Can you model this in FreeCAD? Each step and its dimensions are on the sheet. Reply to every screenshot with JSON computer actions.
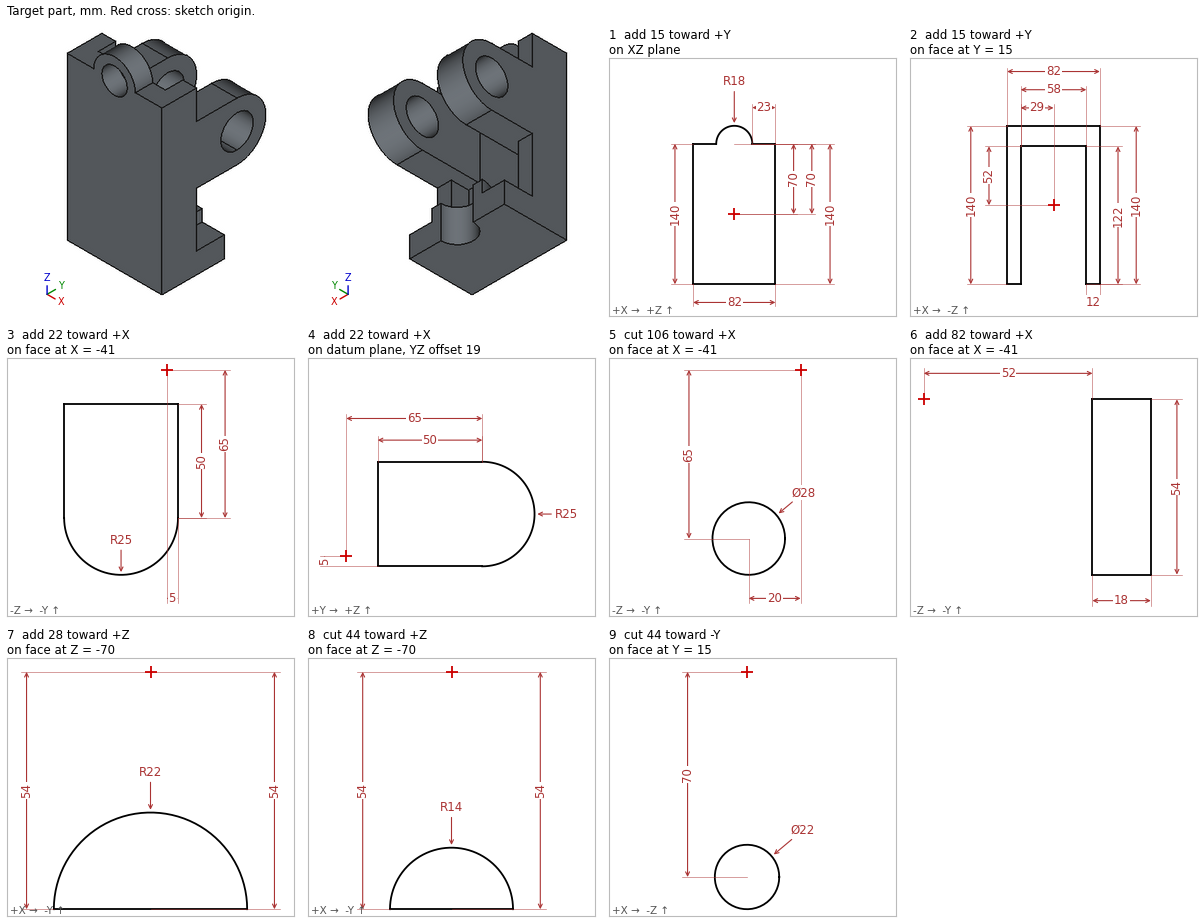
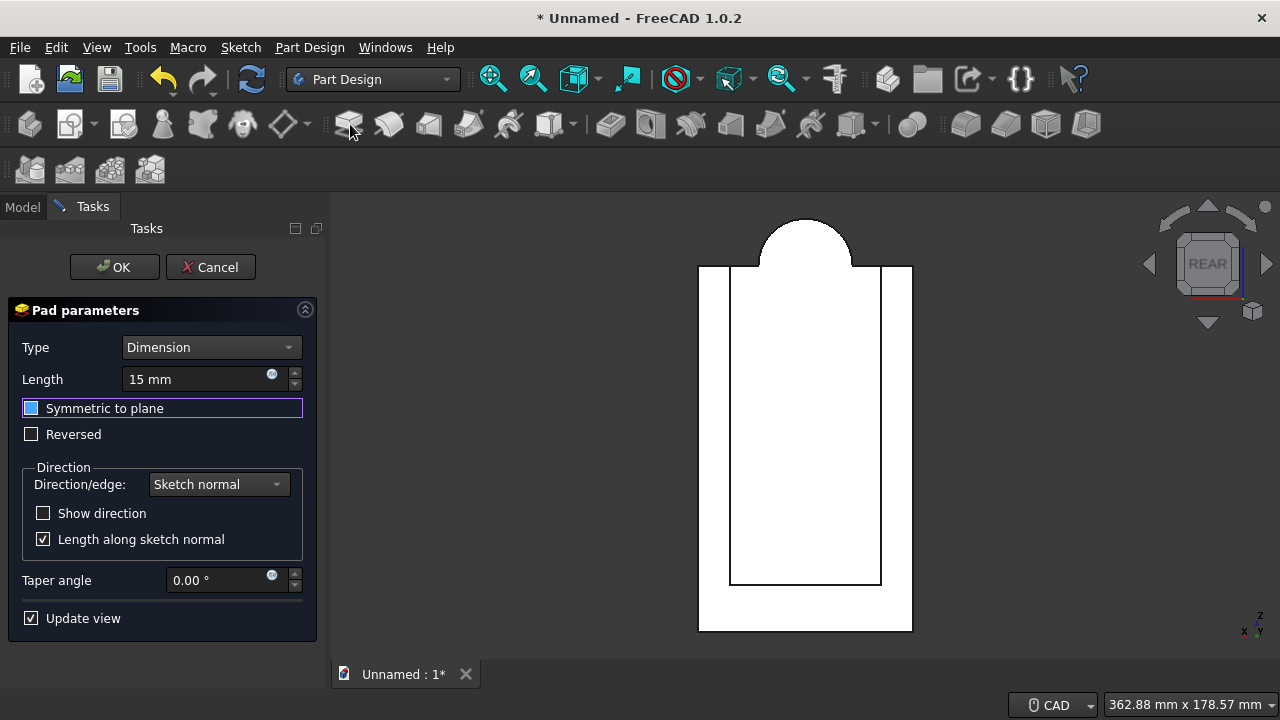
{"action": "left_click", "coordinate": [115, 267]}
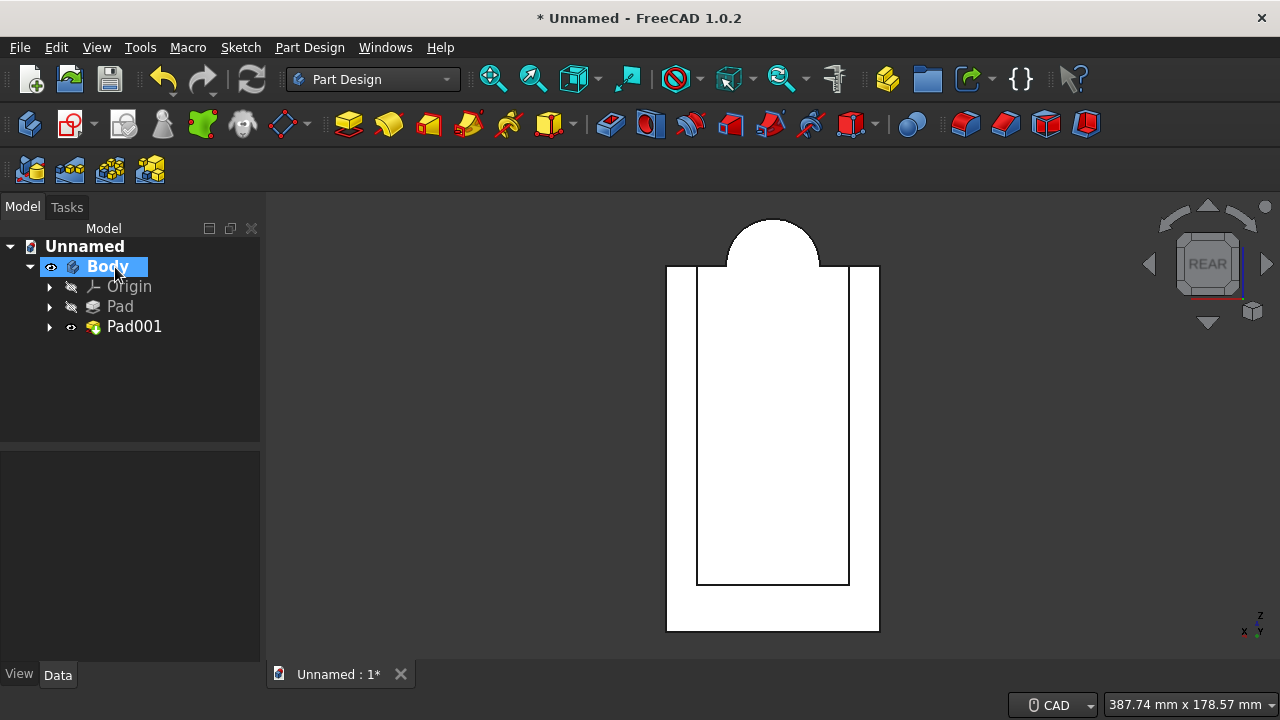
{"action": "key", "text": "6"}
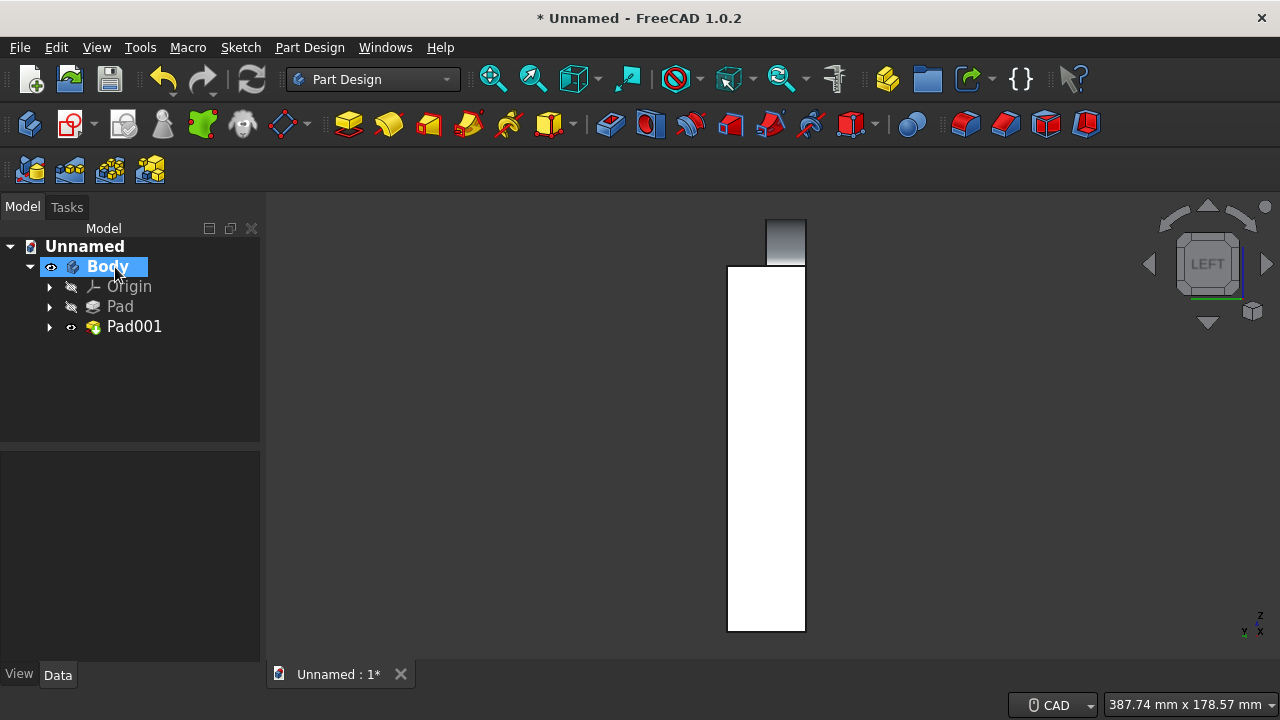
{"action": "left_click", "coordinate": [766, 553]}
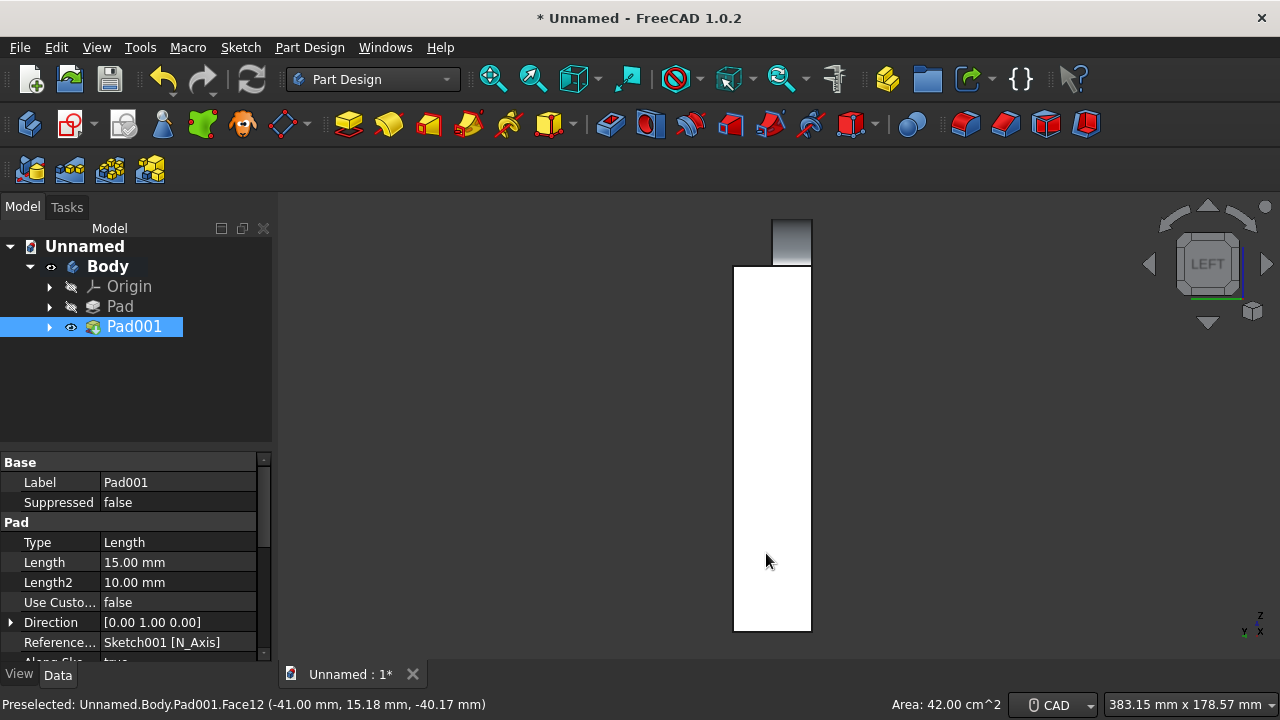
{"action": "left_click", "coordinate": [70, 124]}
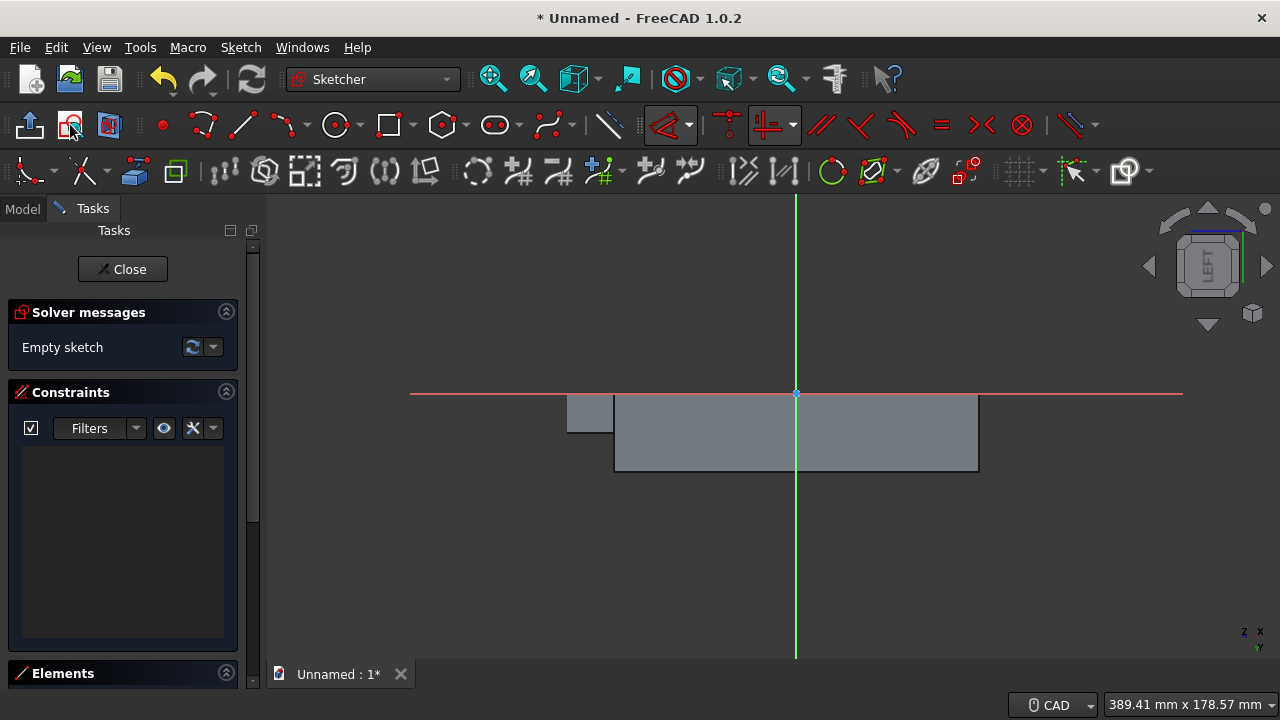
{"action": "scroll", "coordinate": [525, 222], "scroll_direction": "down", "scroll_amount": 1}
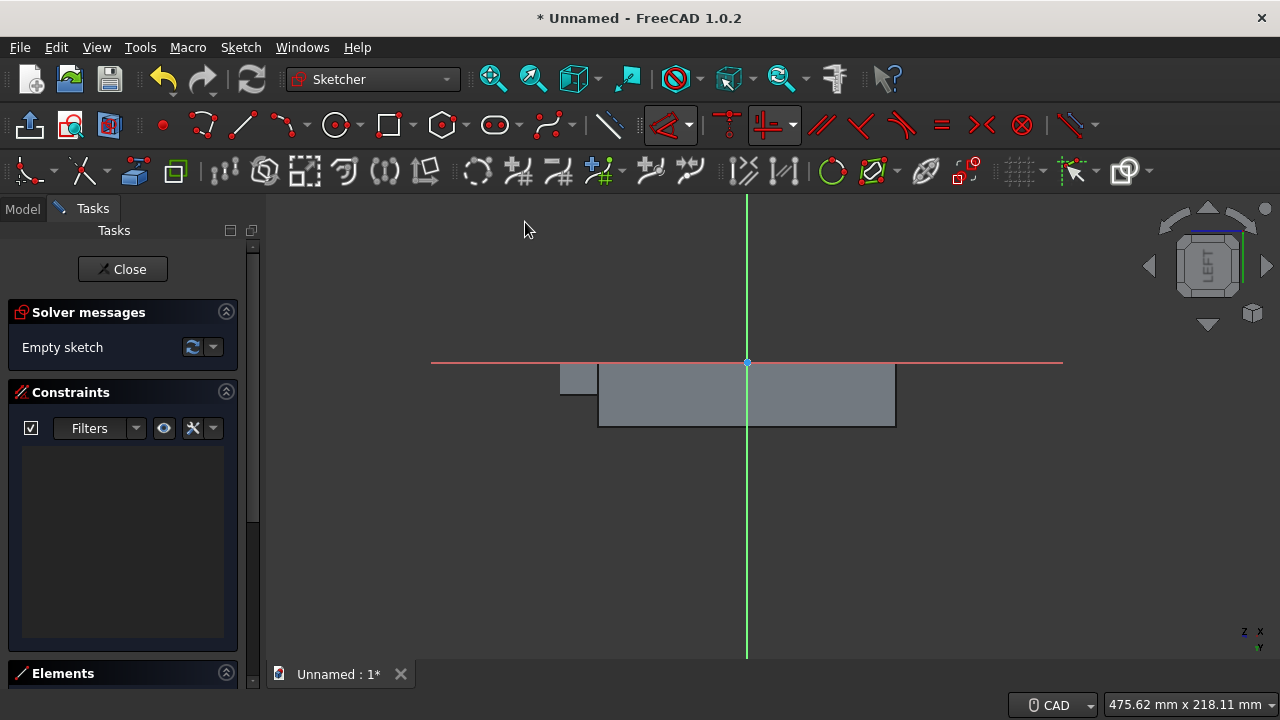
{"action": "scroll", "coordinate": [705, 524], "scroll_direction": "up", "scroll_amount": 2}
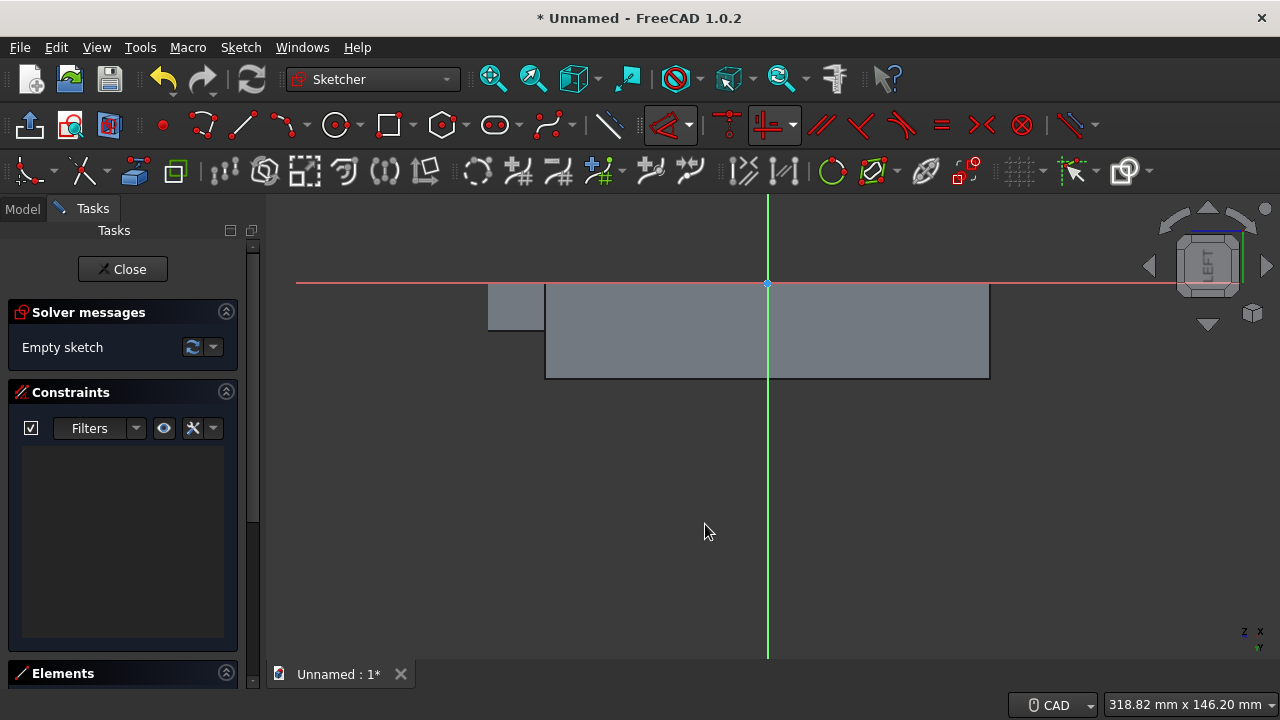
{"action": "left_click", "coordinate": [204, 126]}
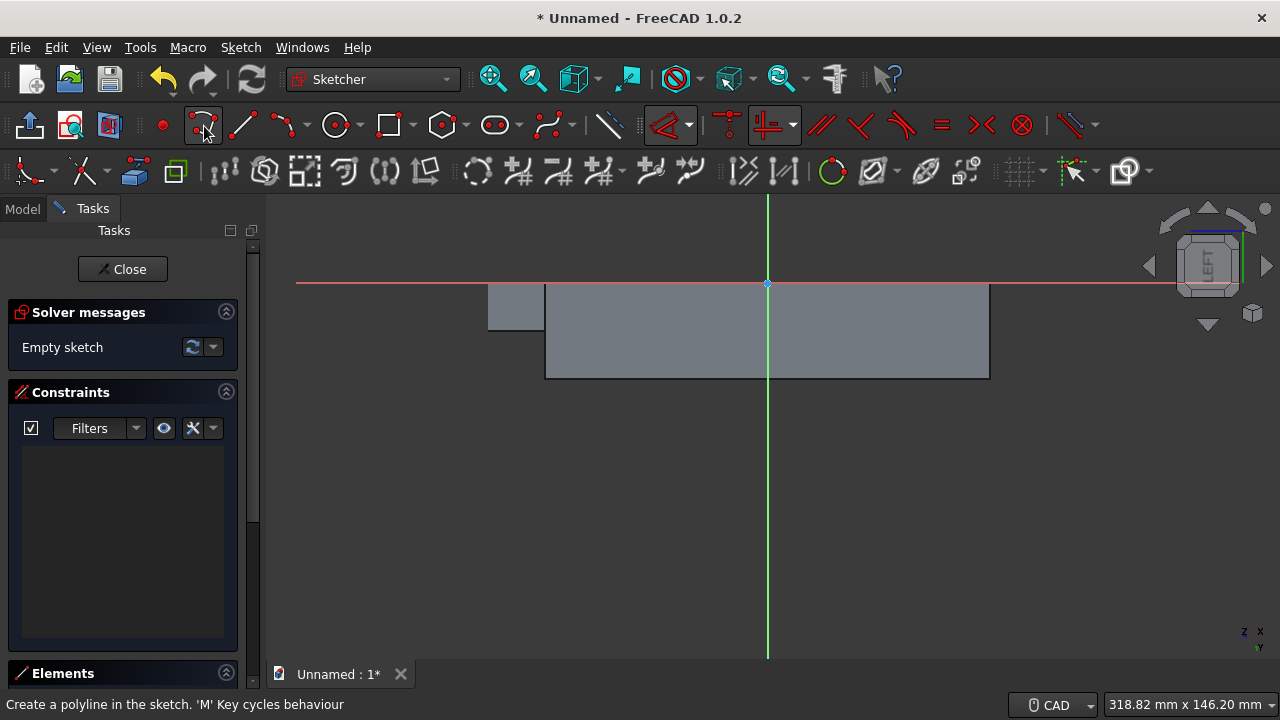
{"action": "left_click", "coordinate": [784, 490]}
{"action": "left_click", "coordinate": [784, 331]}
{"action": "left_click", "coordinate": [625, 331]}
{"action": "left_click", "coordinate": [625, 490]}
{"action": "right_click", "coordinate": [625, 490]}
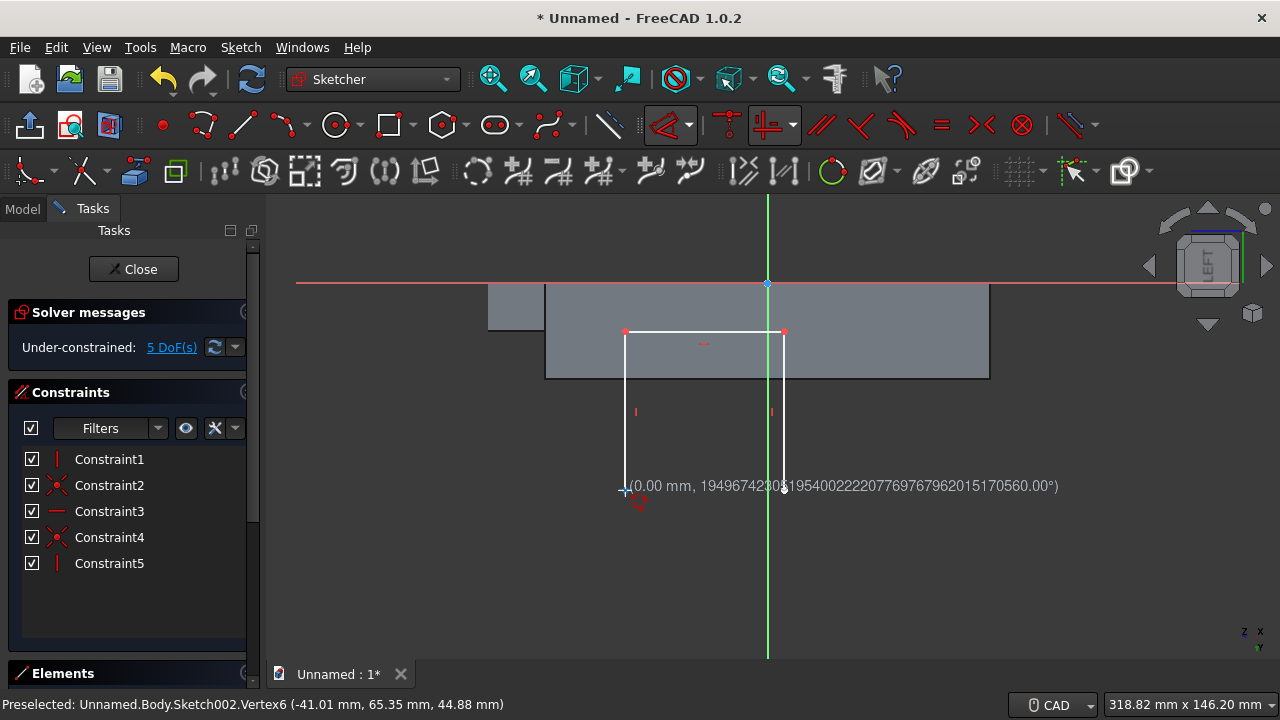
{"action": "key", "text": "g 3 a"}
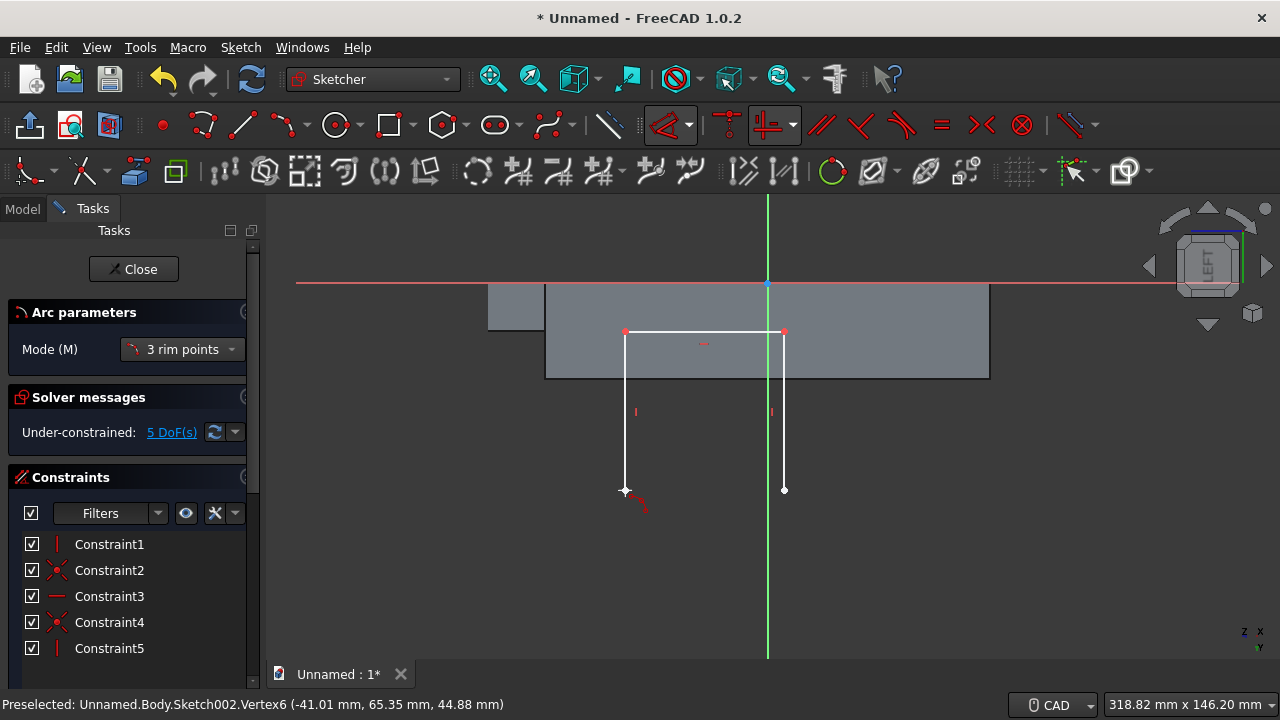
{"action": "left_click", "coordinate": [625, 491]}
{"action": "left_click", "coordinate": [784, 491]}
{"action": "left_click", "coordinate": [704, 569]}
{"action": "key", "text": "Escape"}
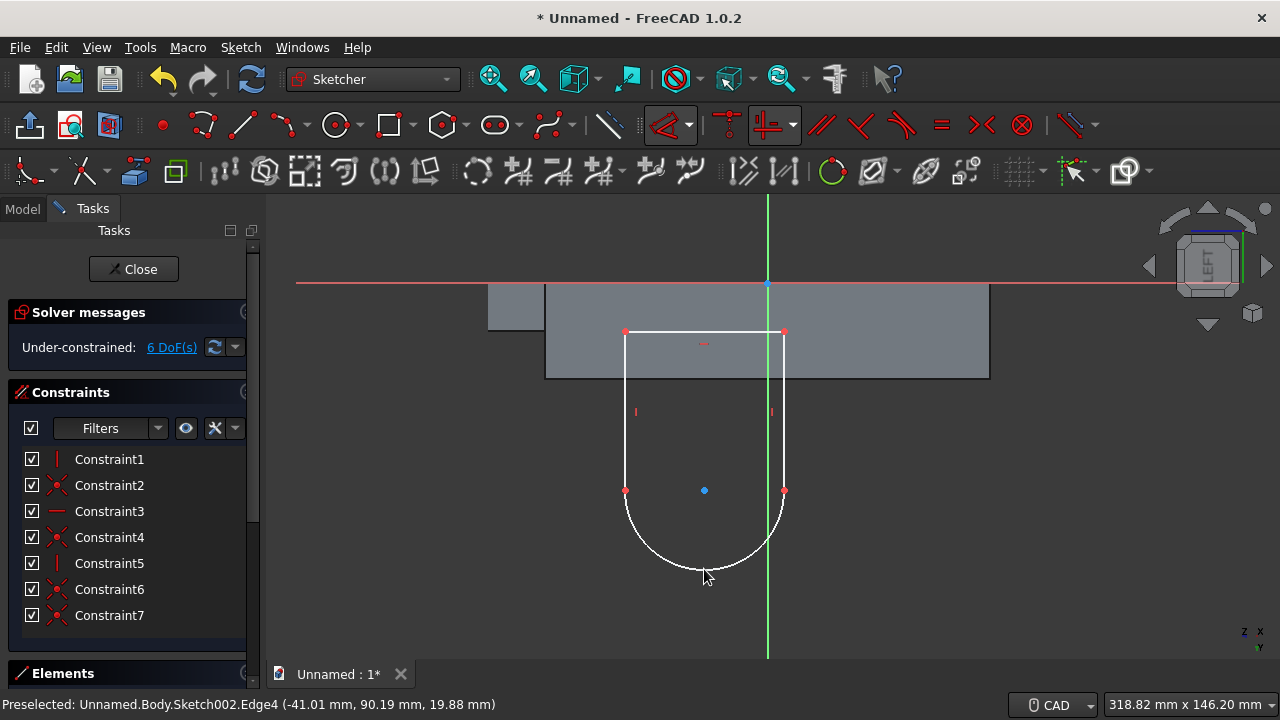
{"action": "left_click", "coordinate": [784, 443]}